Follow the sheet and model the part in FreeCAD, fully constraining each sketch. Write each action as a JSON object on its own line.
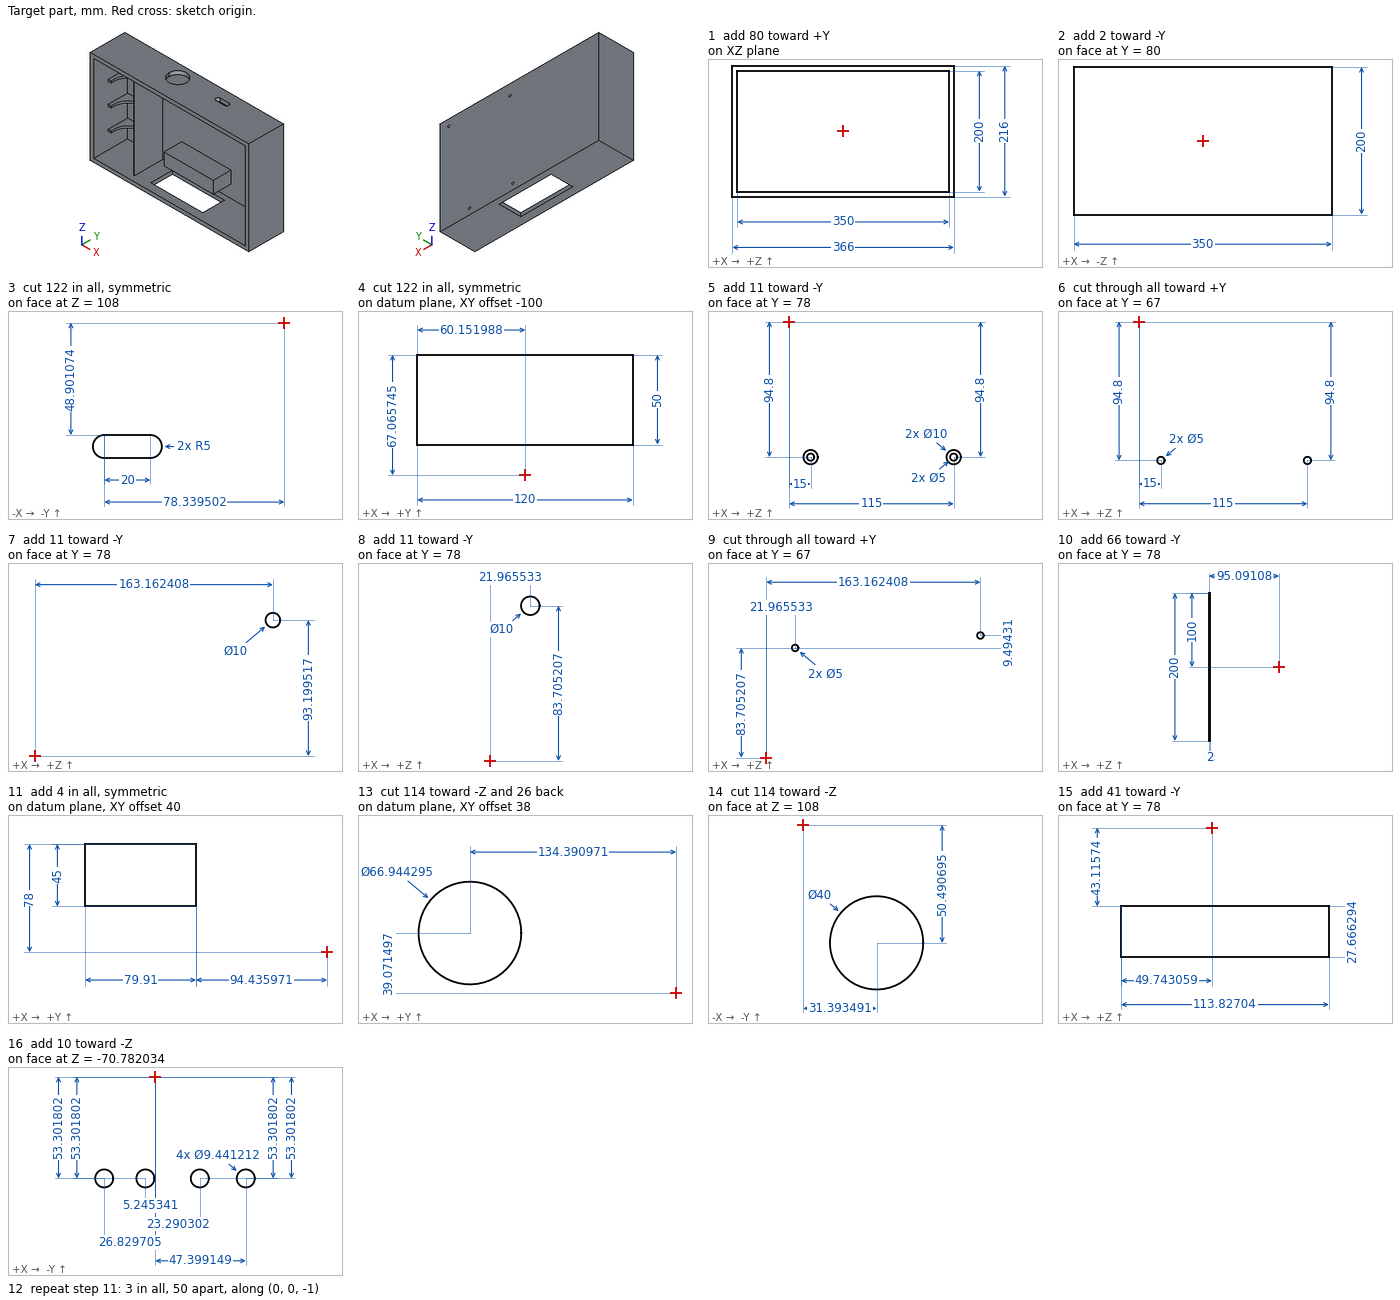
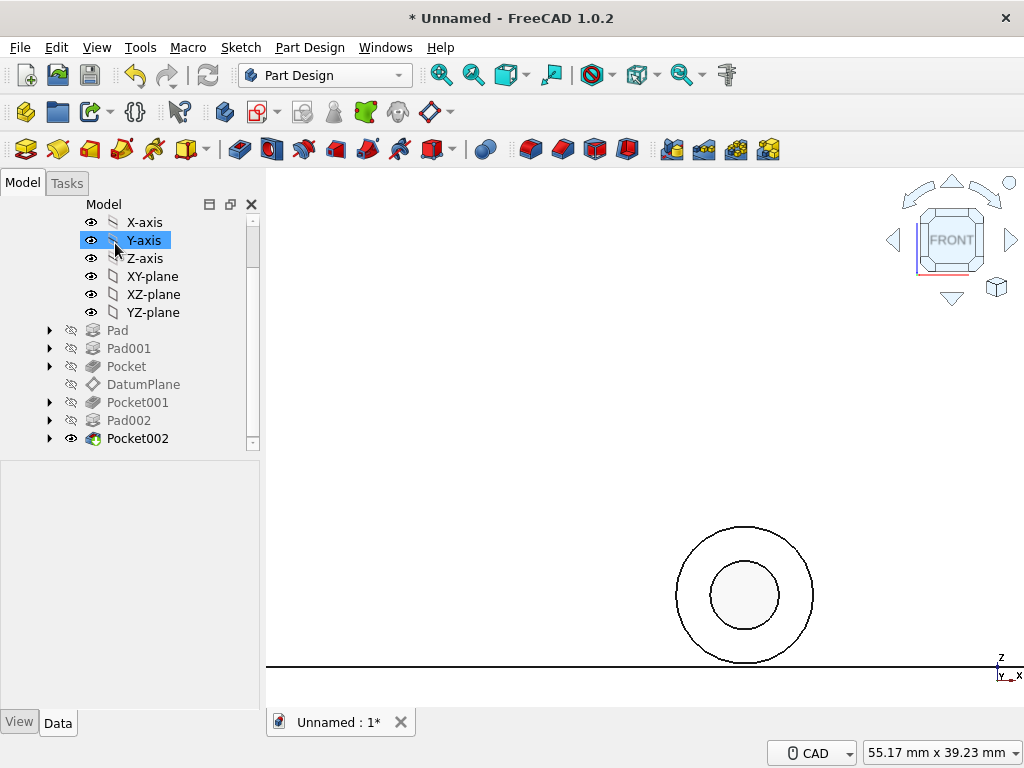
{"action": "key", "text": "v f"}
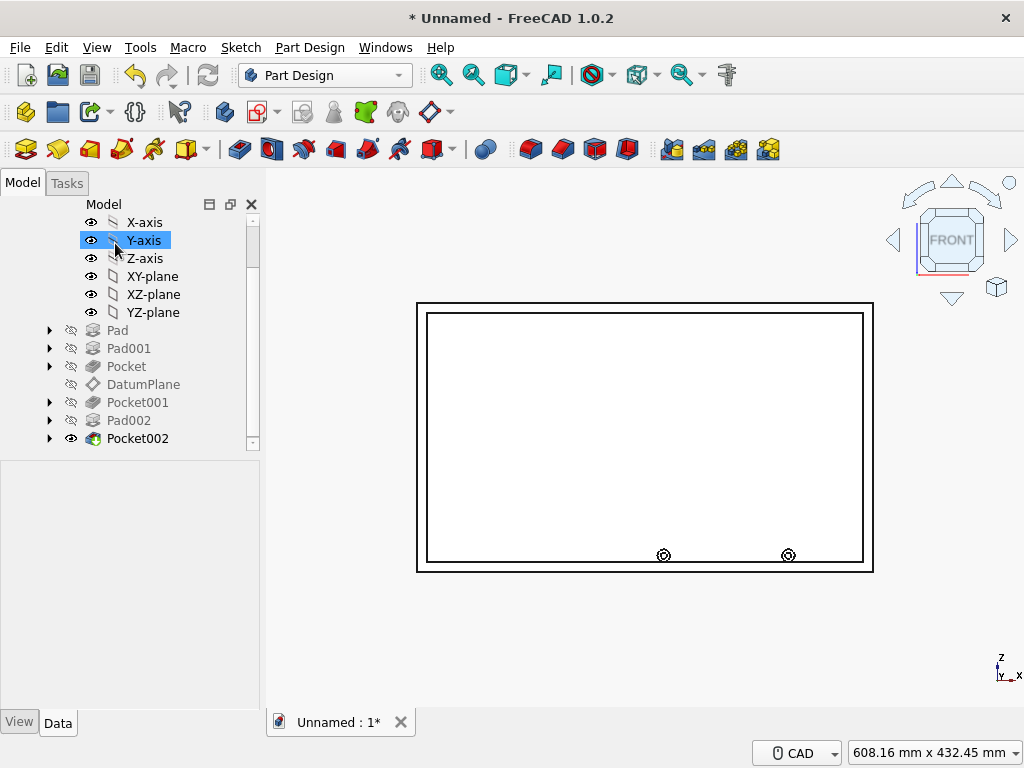
{"action": "left_click", "coordinate": [583, 437]}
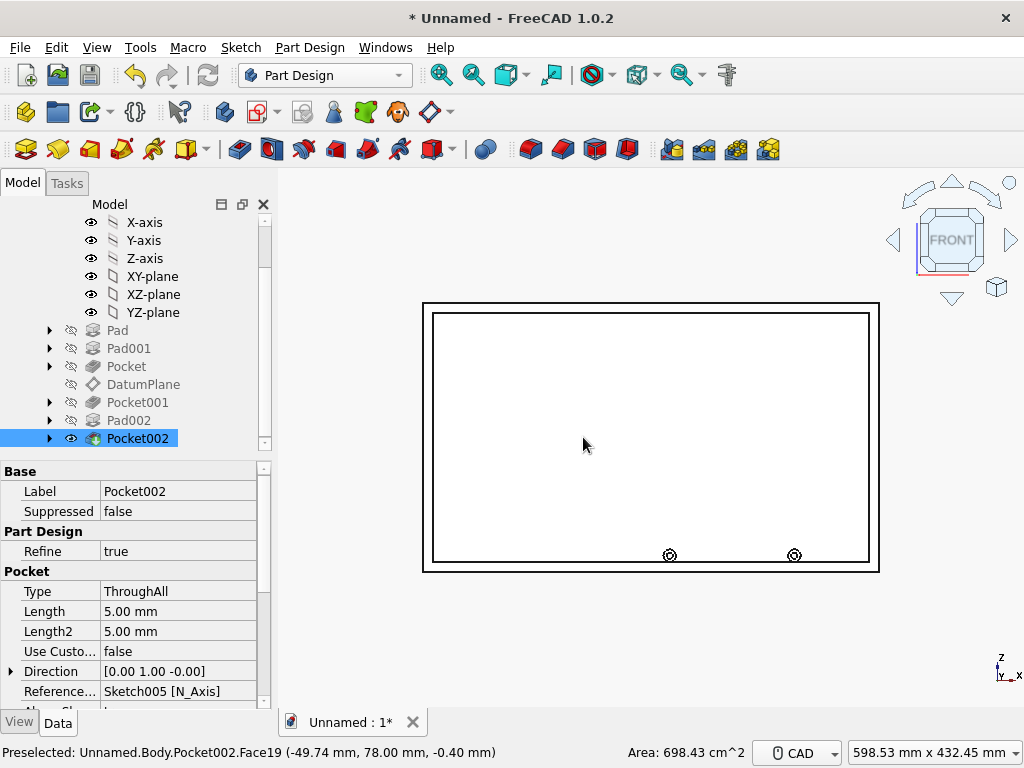
{"action": "left_click", "coordinate": [258, 112]}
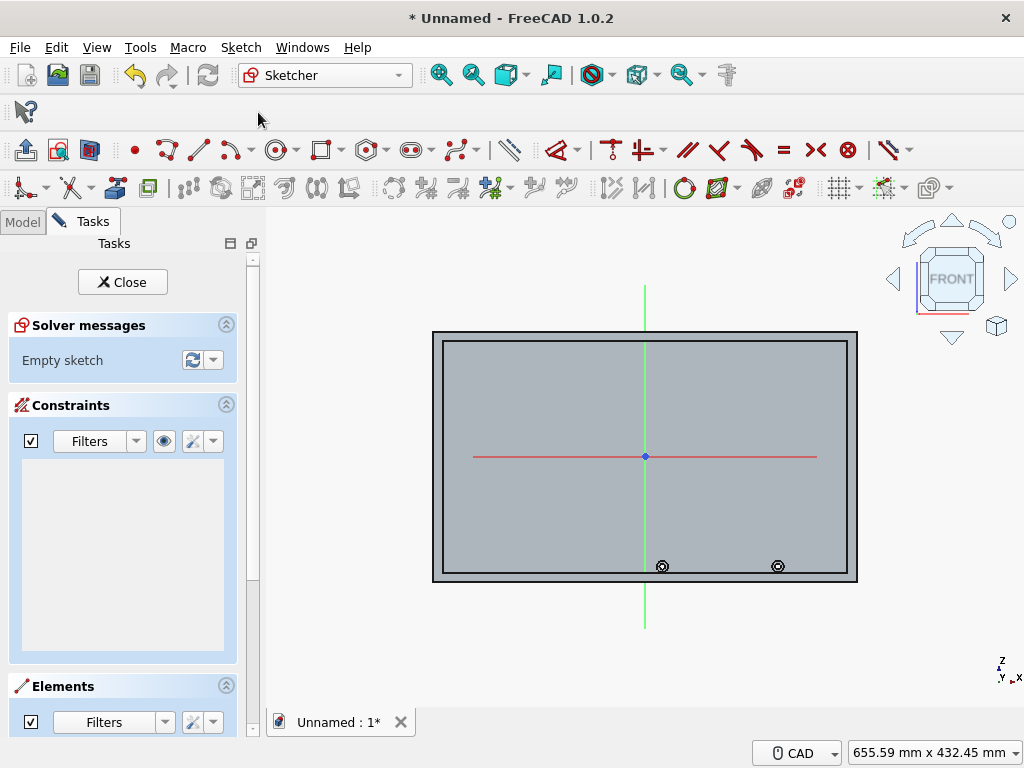
{"action": "key", "text": "q s"}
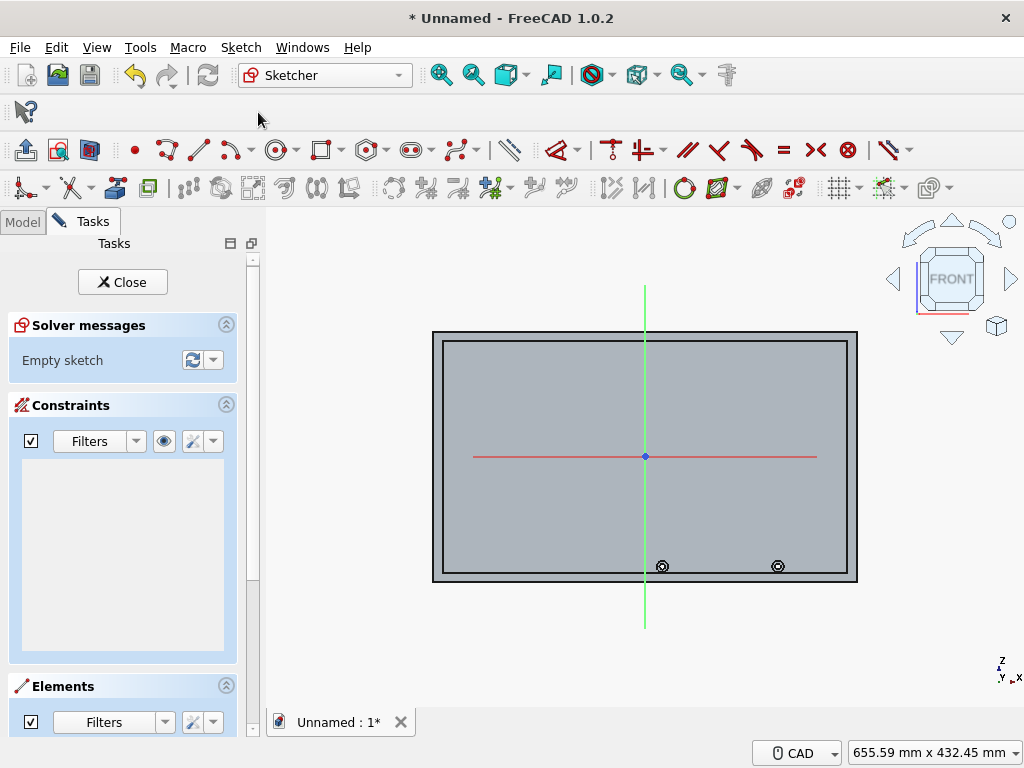
{"action": "scroll", "coordinate": [847, 344], "scroll_direction": "up", "scroll_amount": 15}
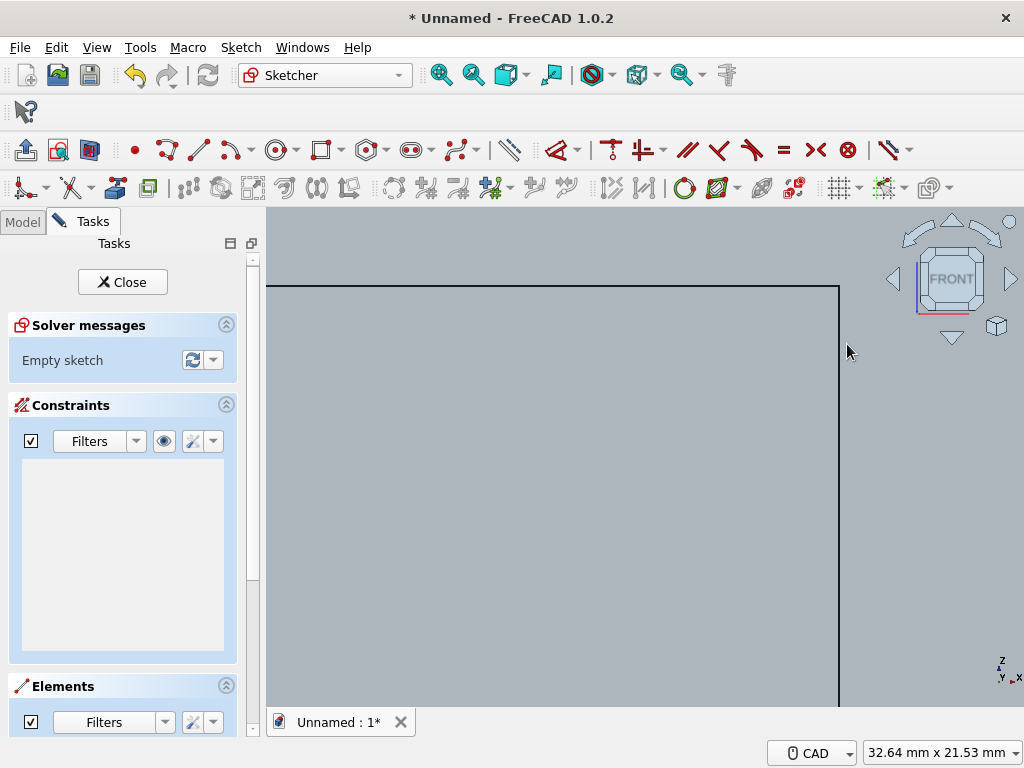
{"action": "key", "text": "g c"}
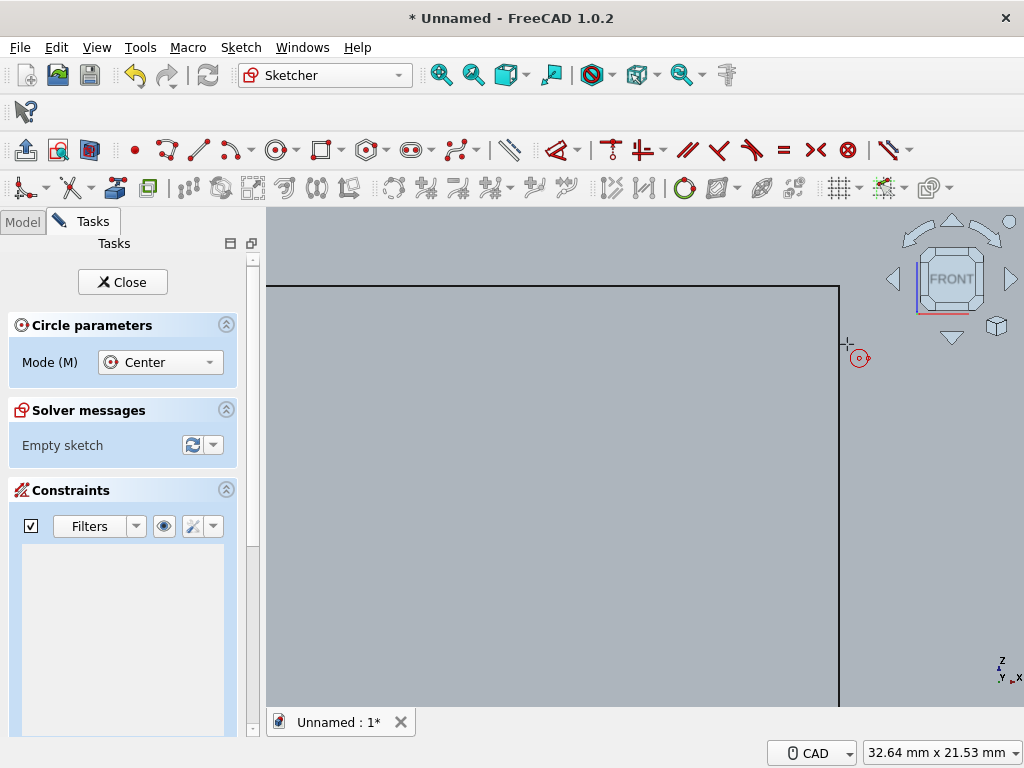
{"action": "left_click", "coordinate": [564, 444]}
{"action": "mouse_move", "coordinate": [646, 362]}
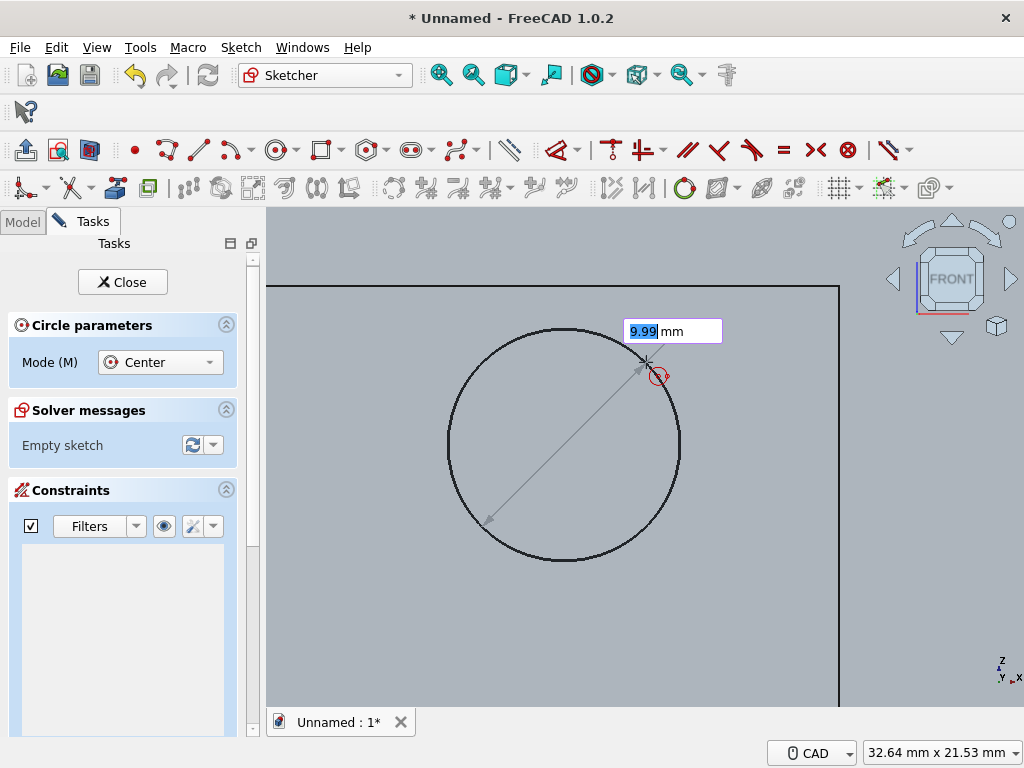
{"action": "type", "text": "10"}
{"action": "key", "text": "Return"}
{"action": "key", "text": "Escape"}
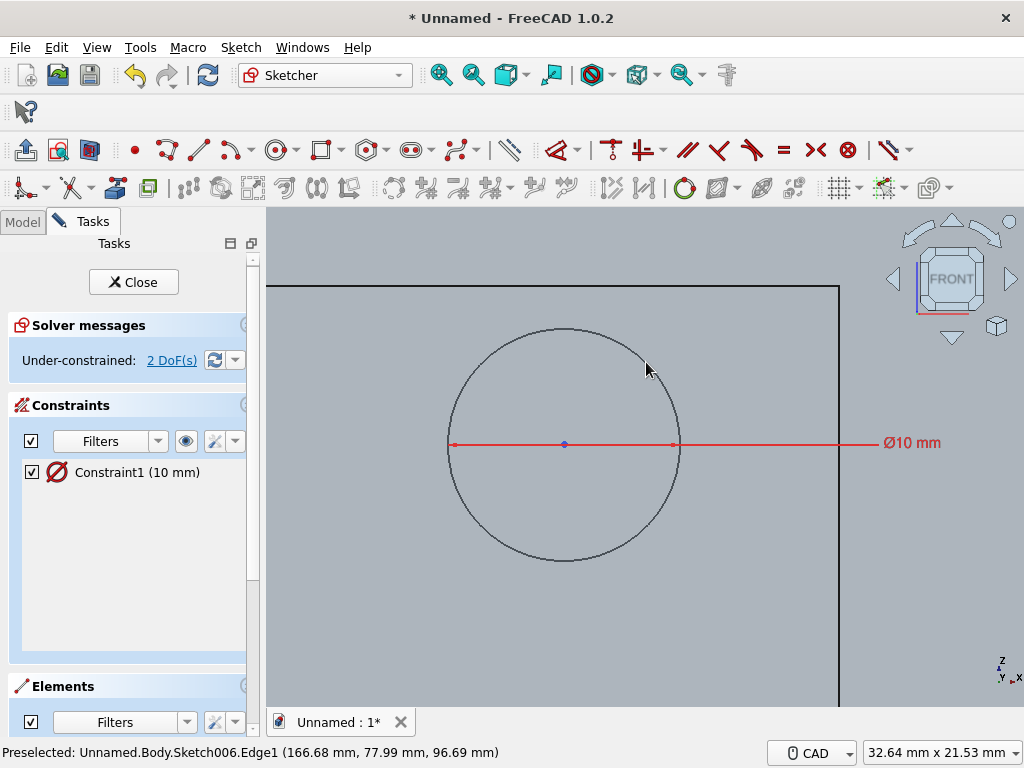
{"action": "left_click", "coordinate": [556, 150]}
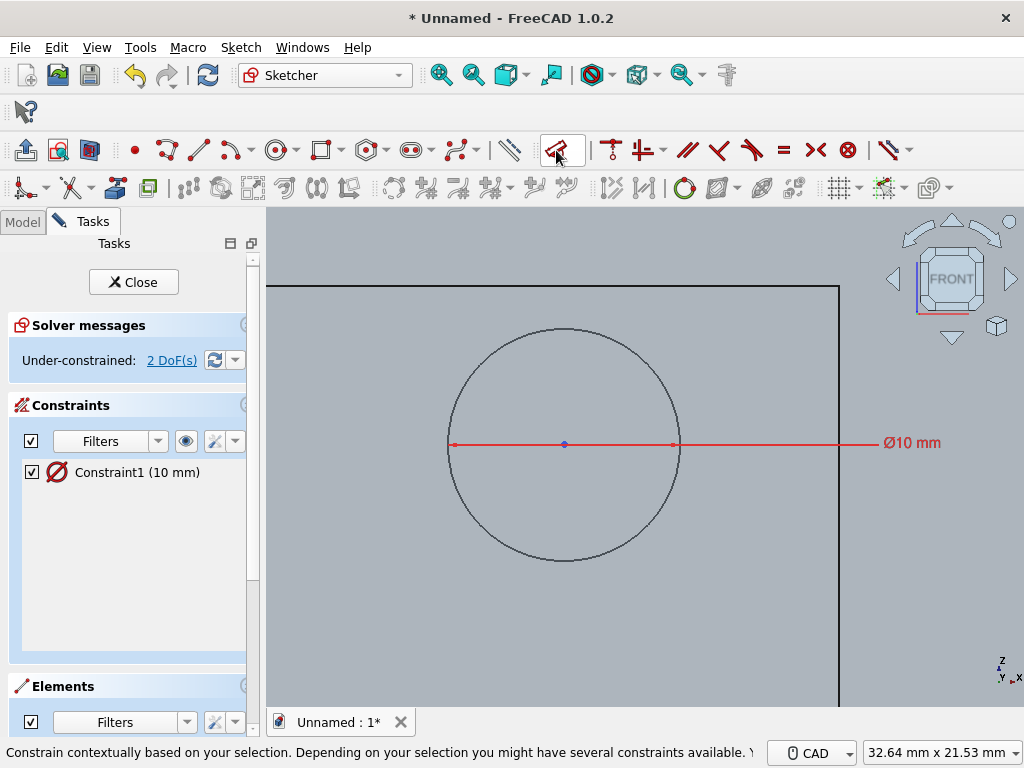
{"action": "left_click", "coordinate": [564, 445]}
{"action": "left_click", "coordinate": [598, 508]}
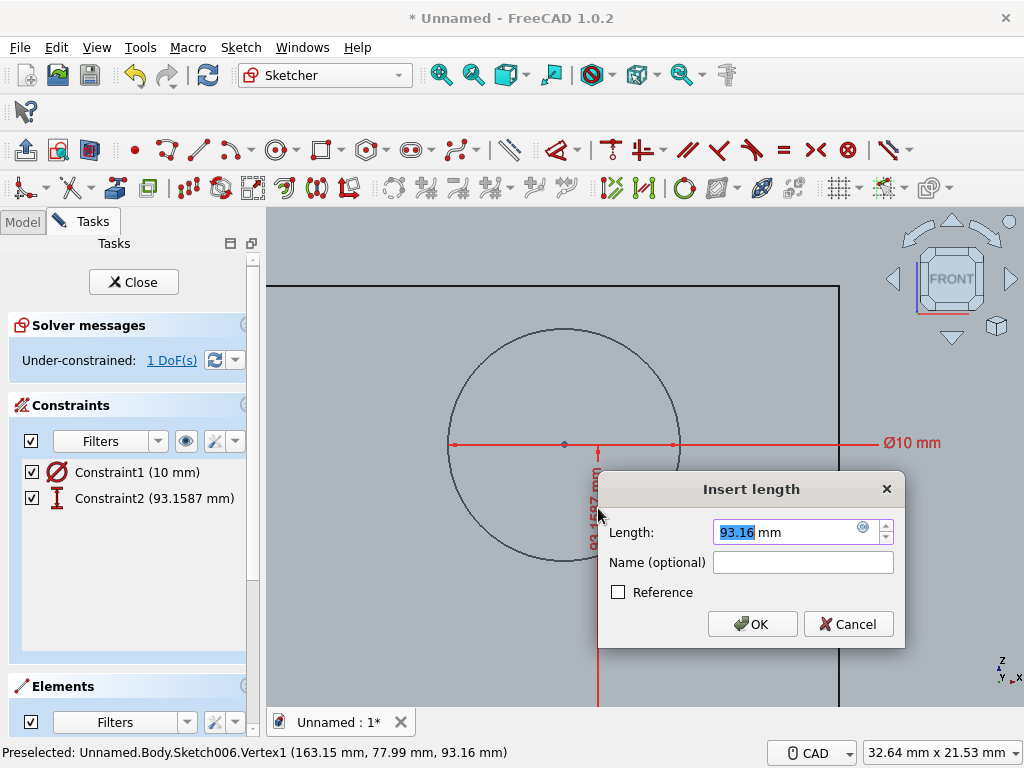
{"action": "type", "text": "93.199517"}
{"action": "key", "text": "Return"}